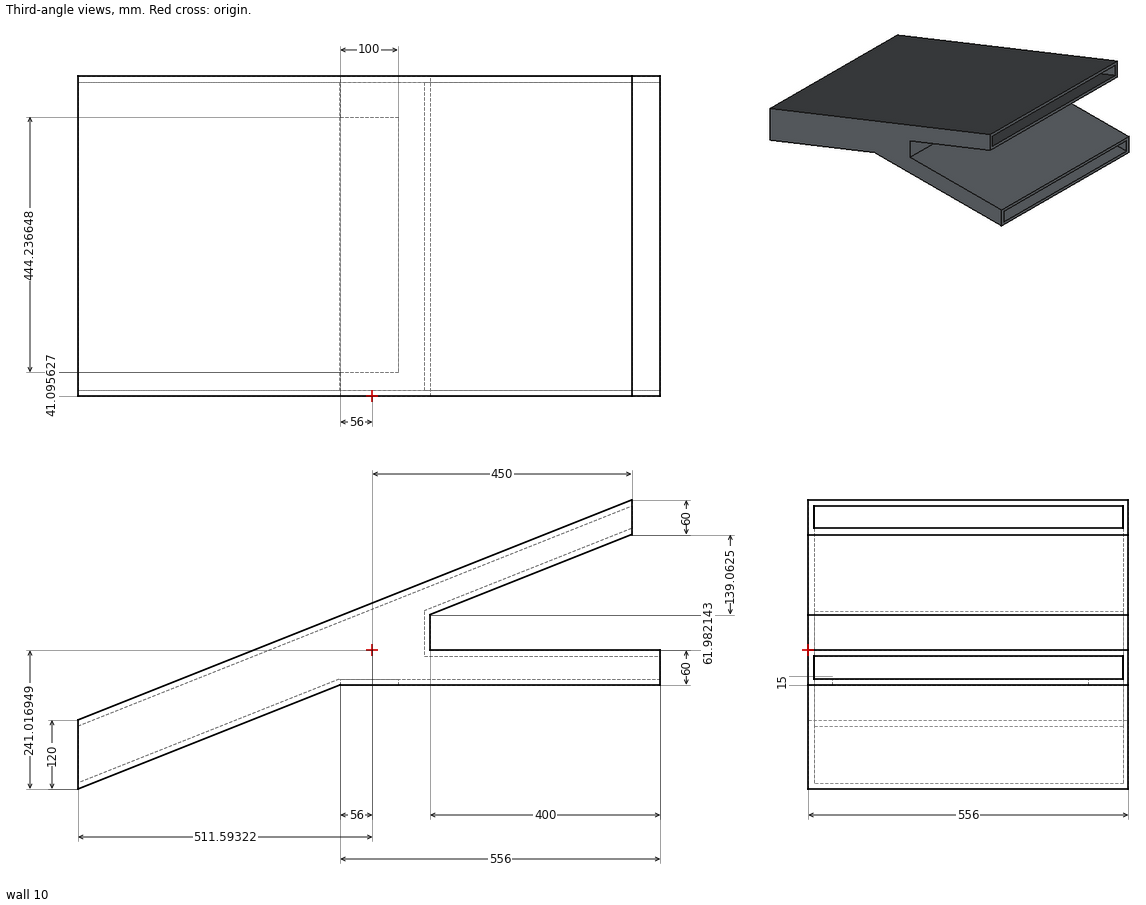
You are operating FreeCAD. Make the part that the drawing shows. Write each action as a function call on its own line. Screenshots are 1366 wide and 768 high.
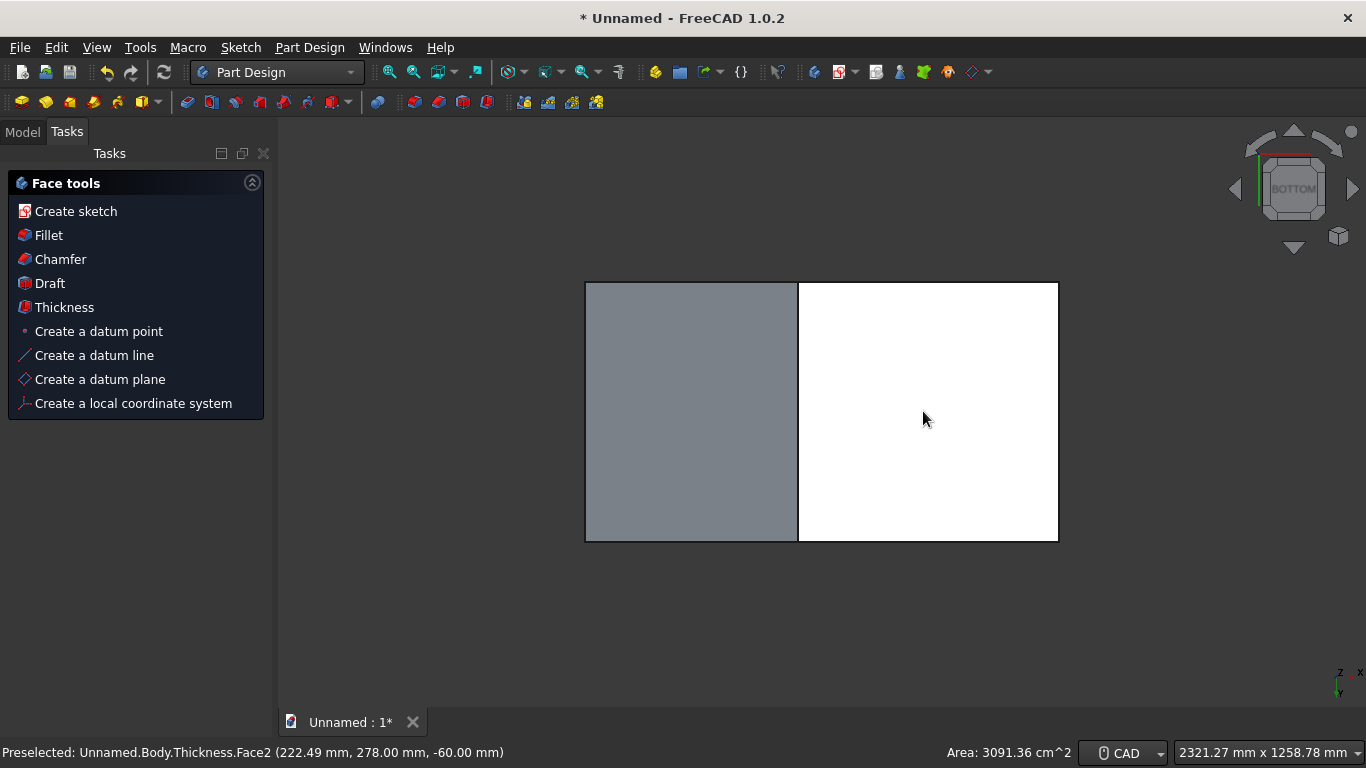
click(840, 72)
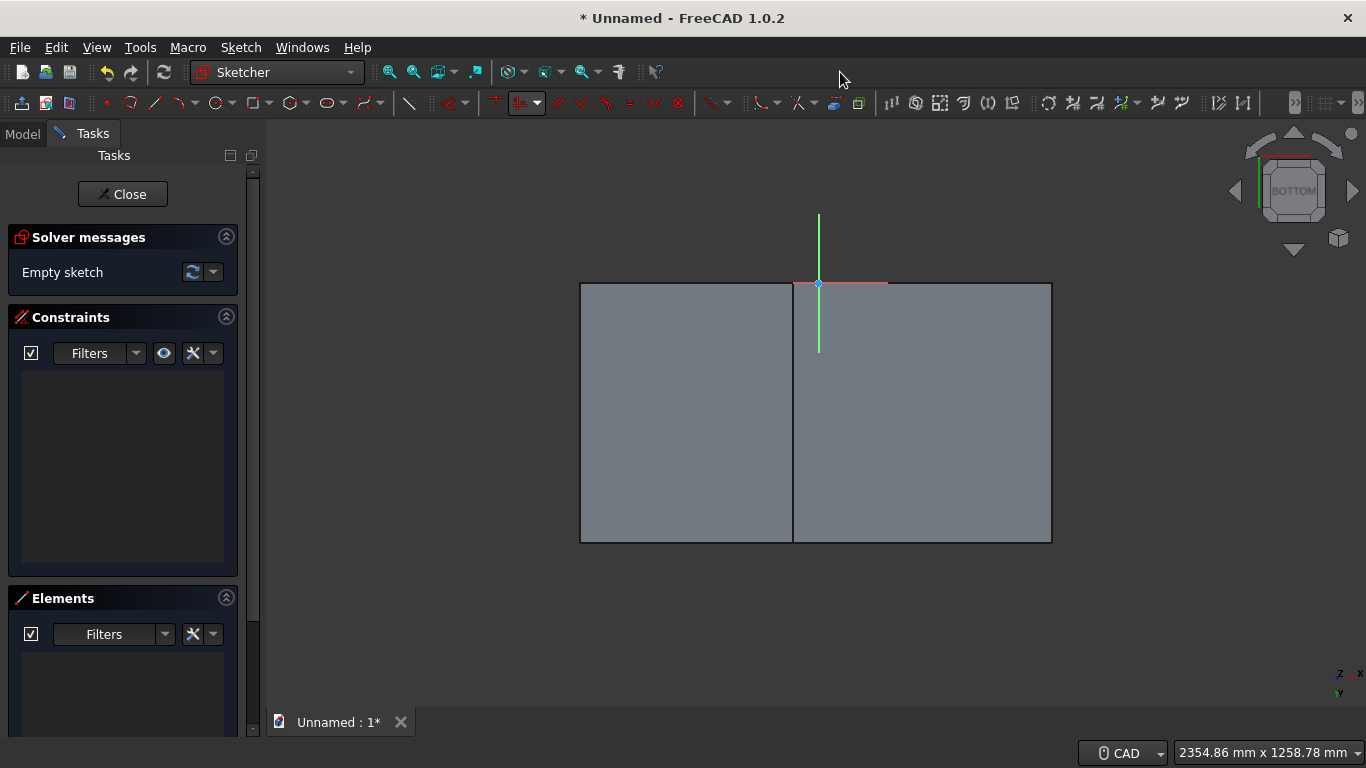
scroll(899, 376, up, 3)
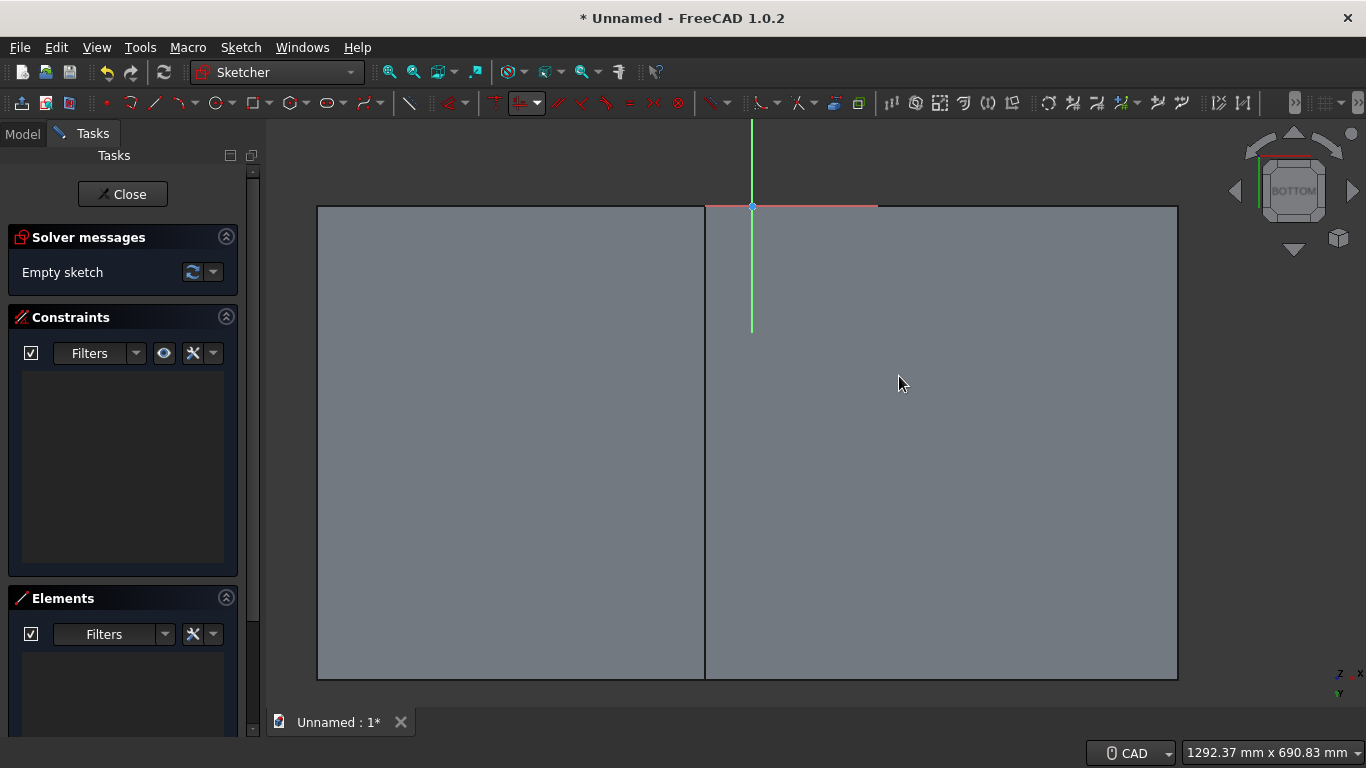
key(g)
key(r)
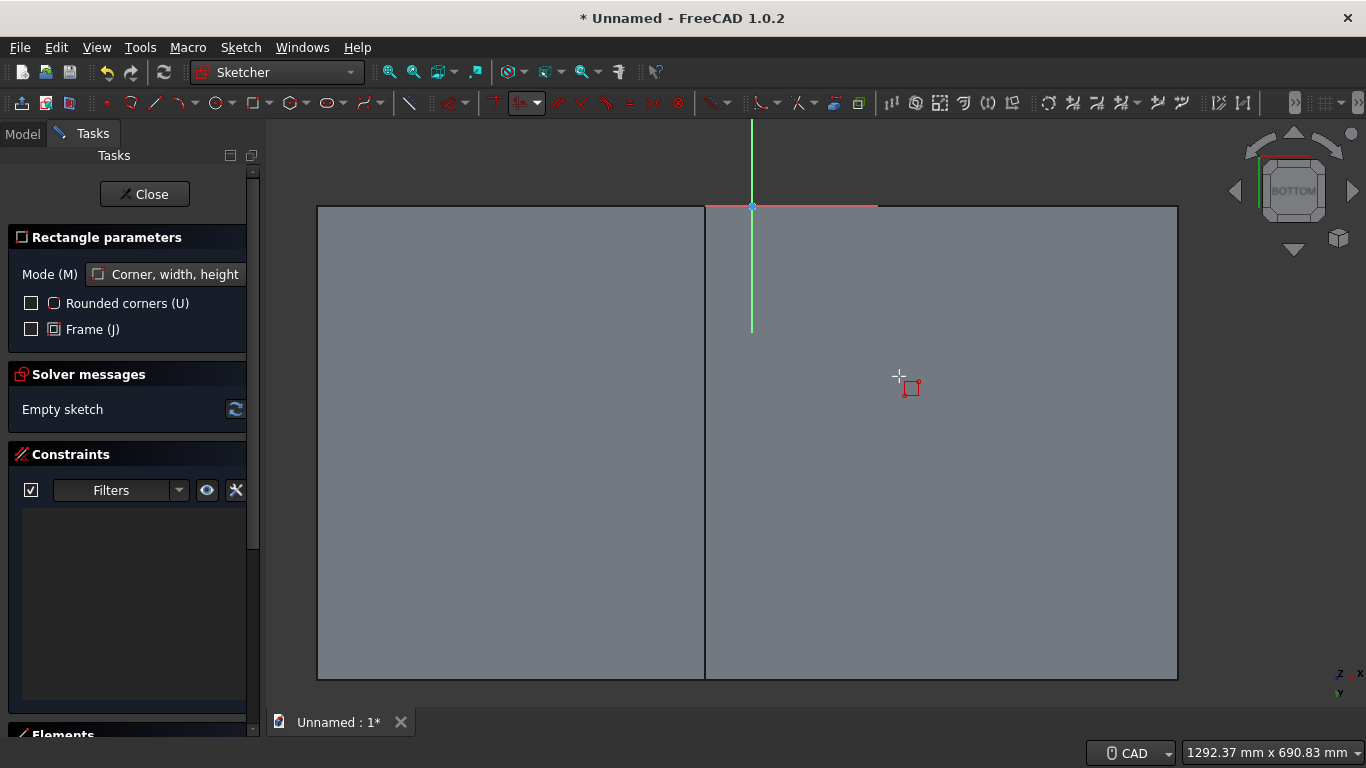
click(705, 241)
click(790, 620)
key(Escape)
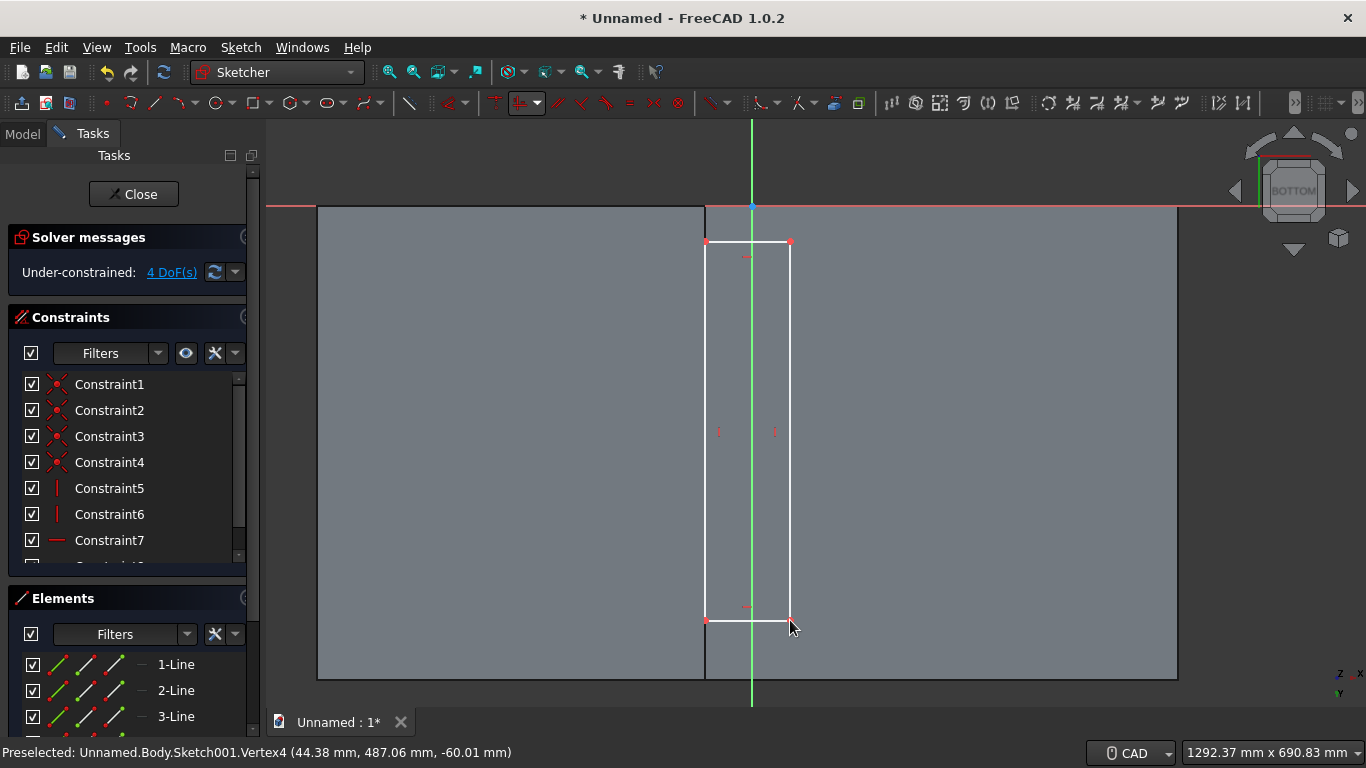
click(448, 104)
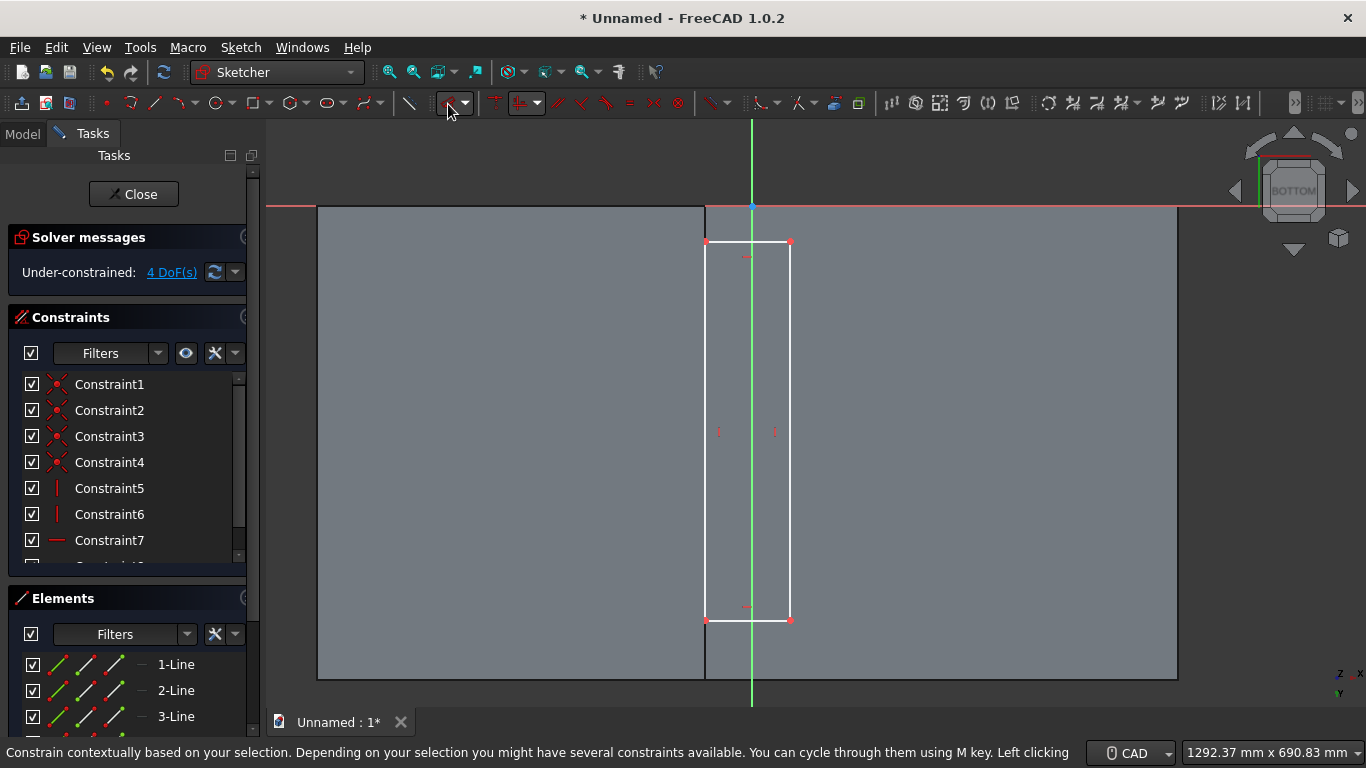
click(731, 621)
click(728, 655)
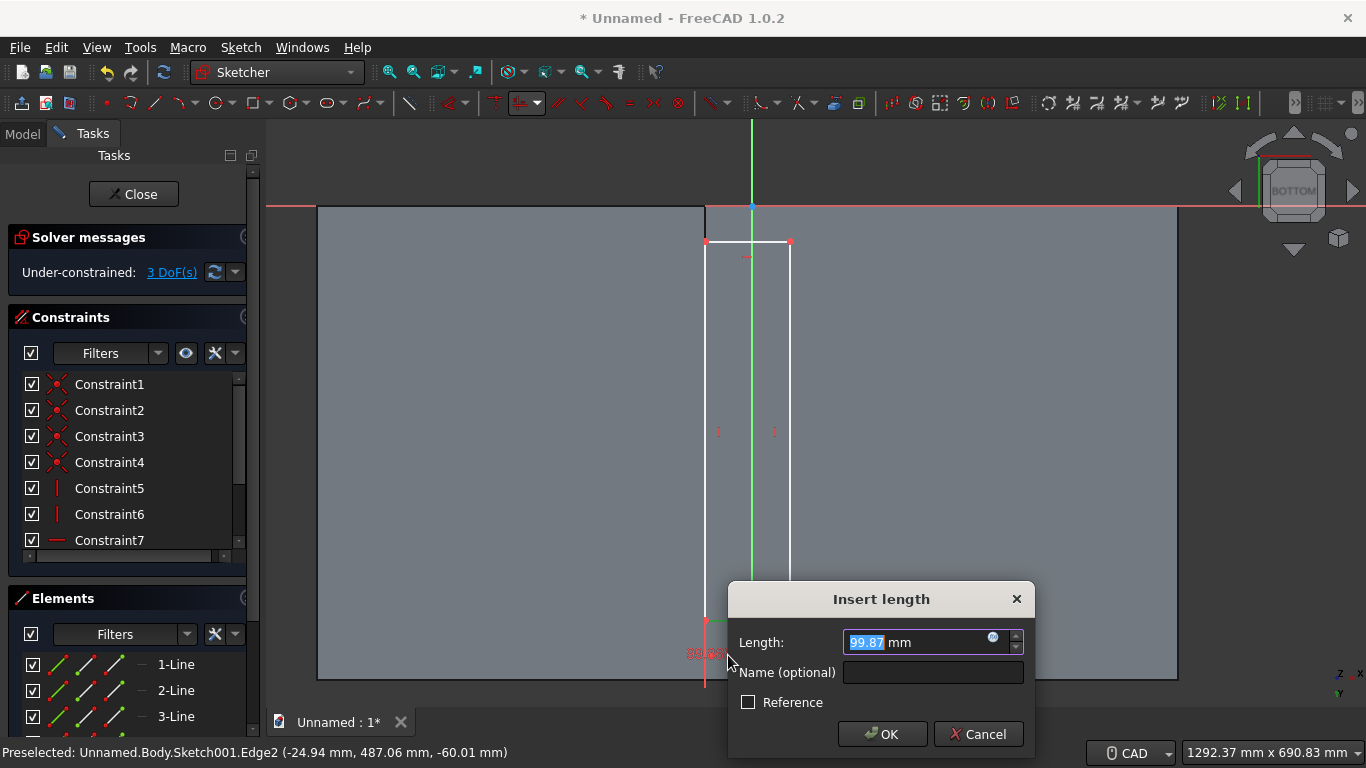
text(100)
key(Return)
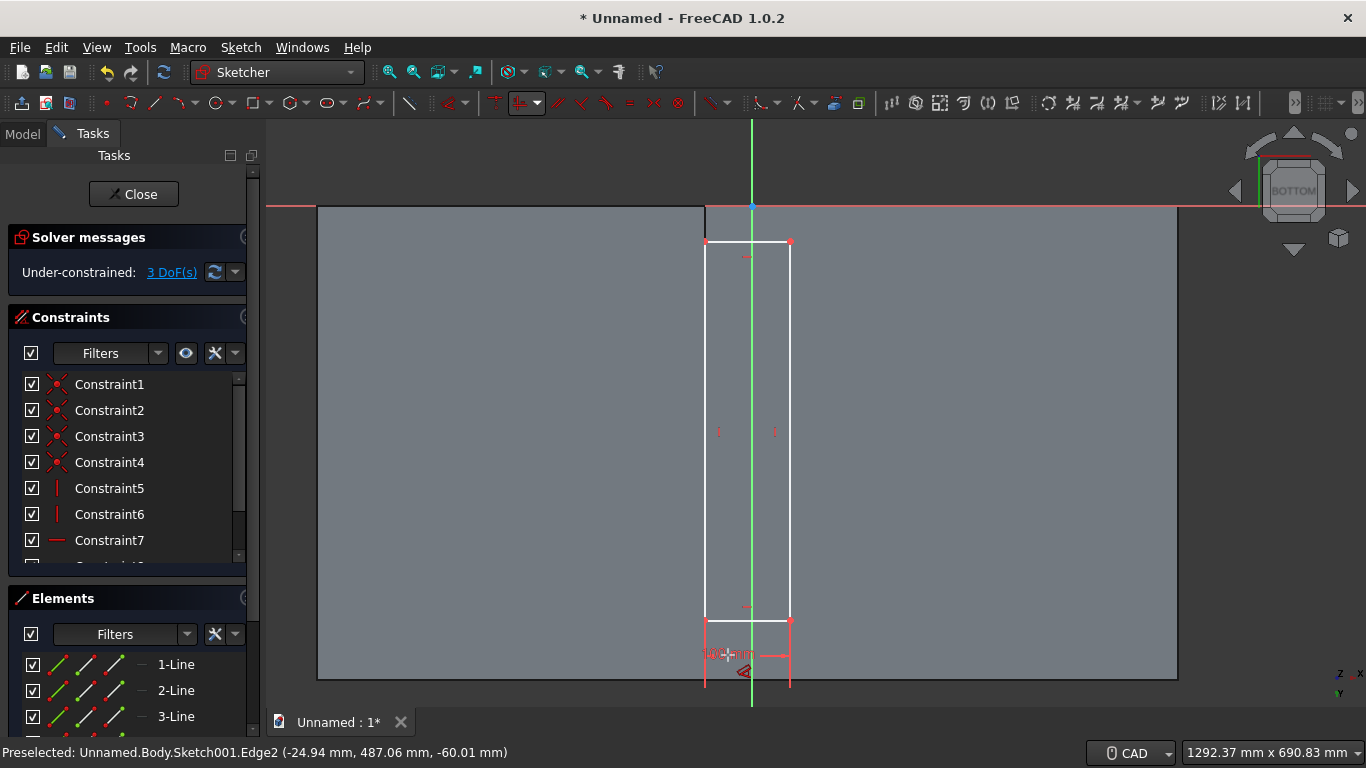
click(705, 242)
click(729, 172)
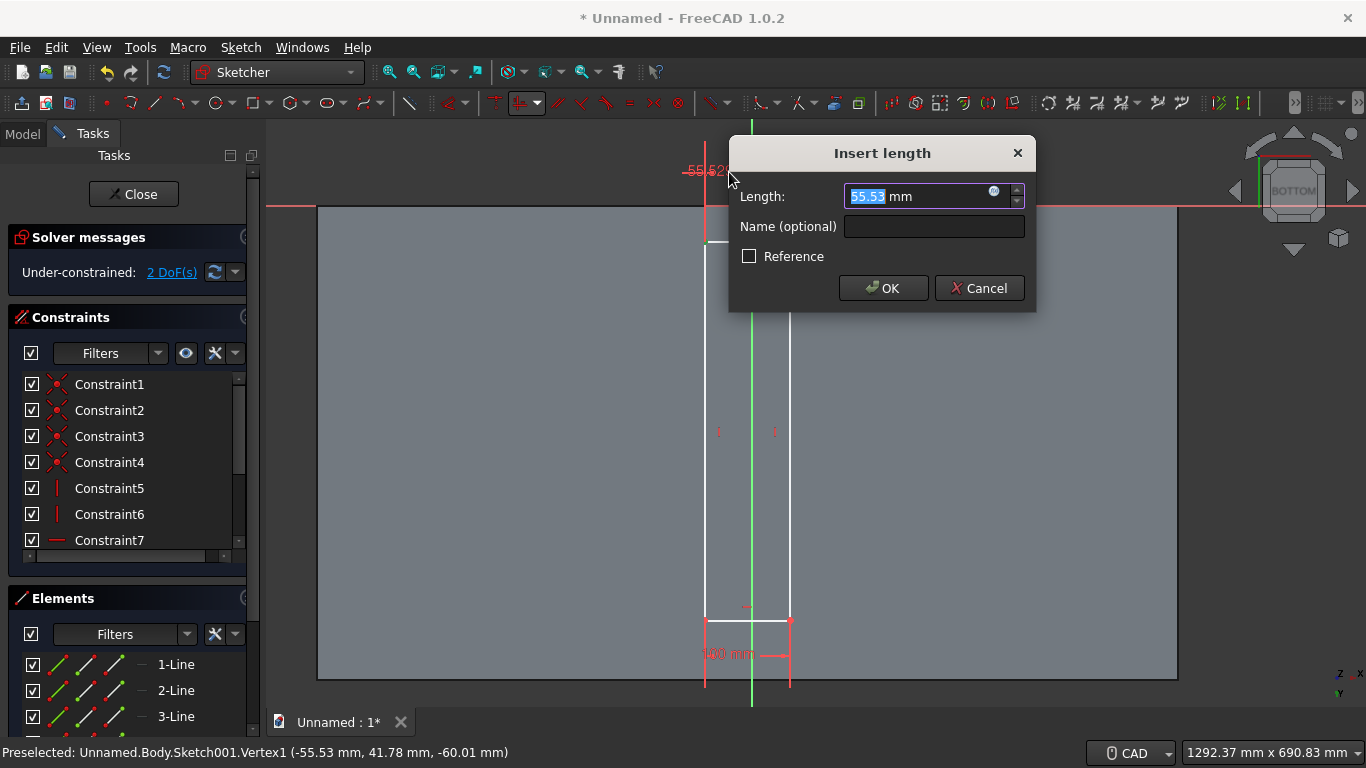
text(56)
key(Return)